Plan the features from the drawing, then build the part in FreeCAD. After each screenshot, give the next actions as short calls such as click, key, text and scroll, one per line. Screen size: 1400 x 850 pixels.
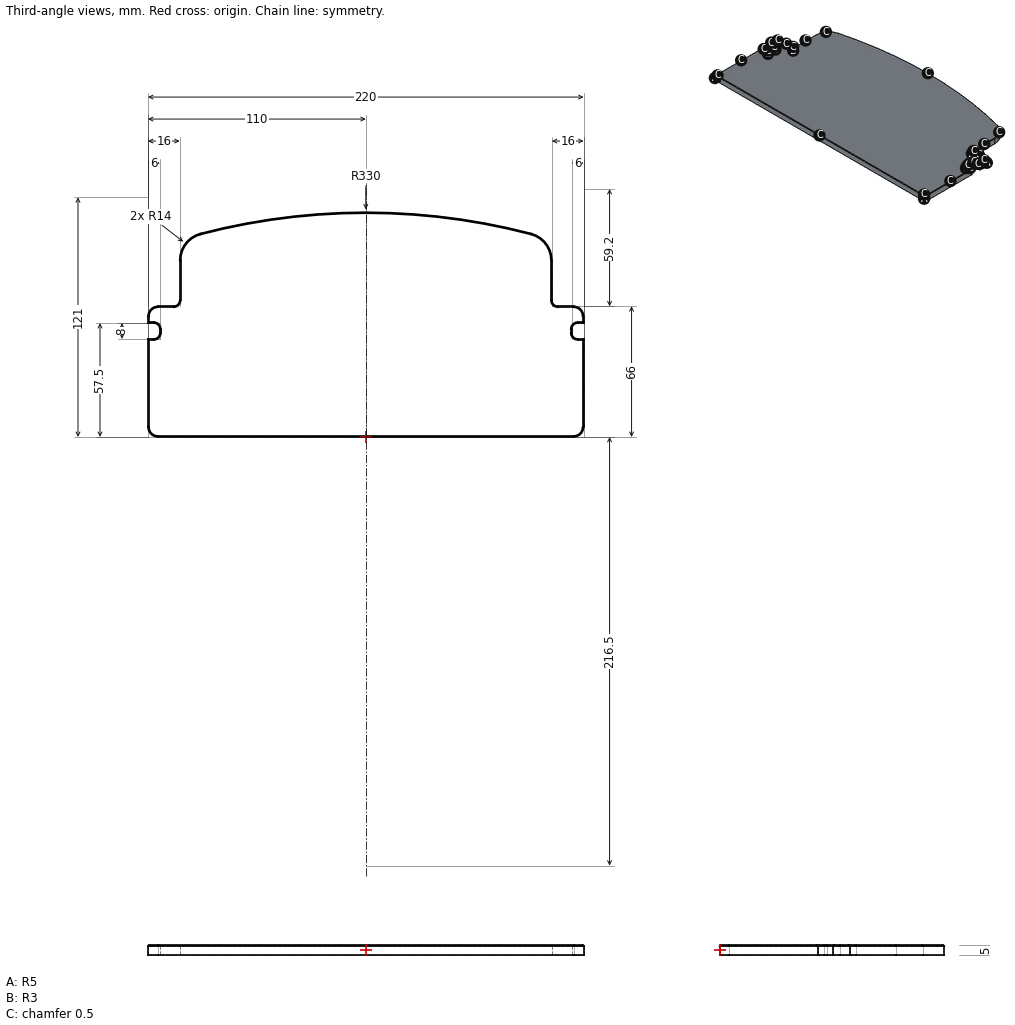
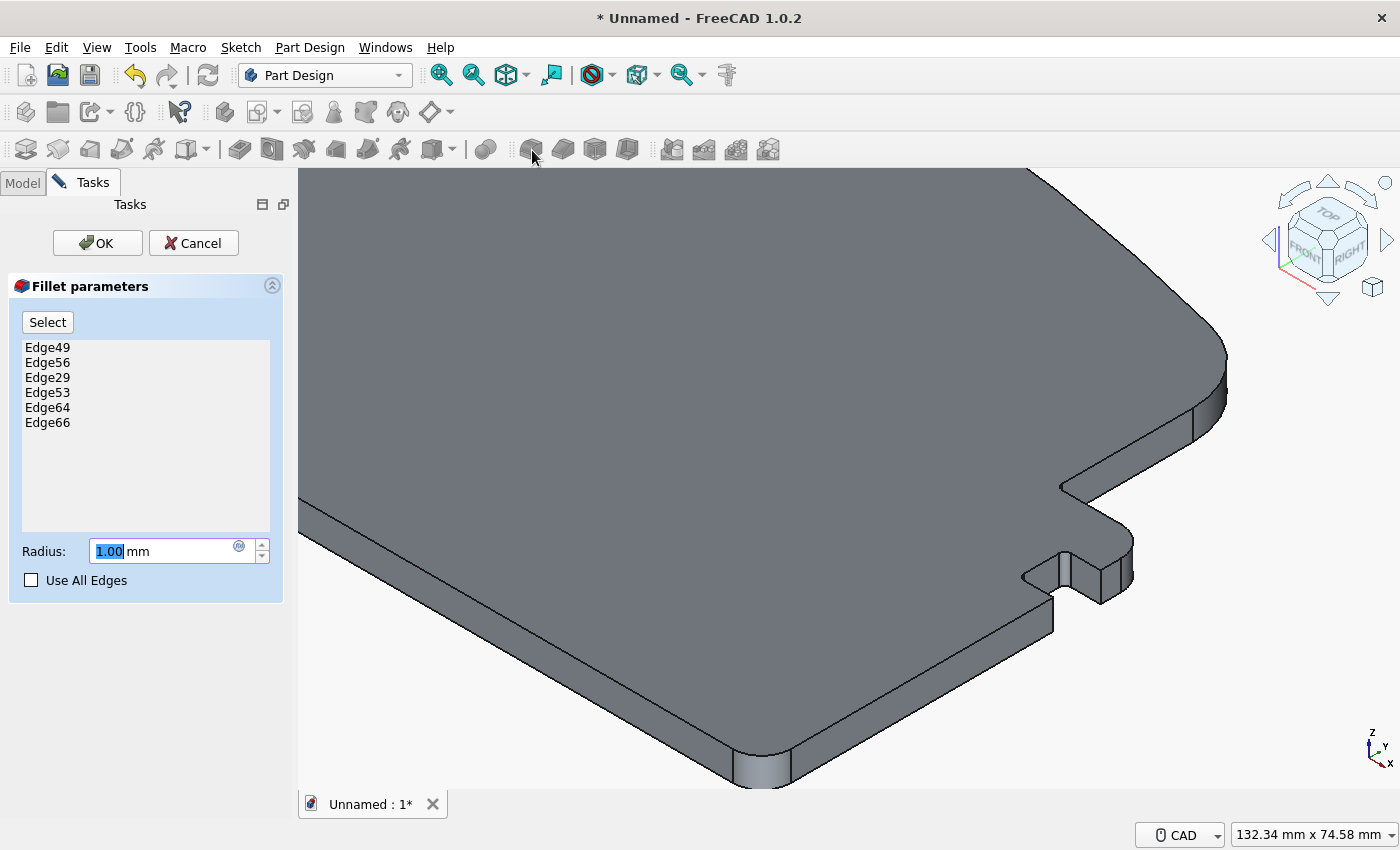
text(3)
key(Tab)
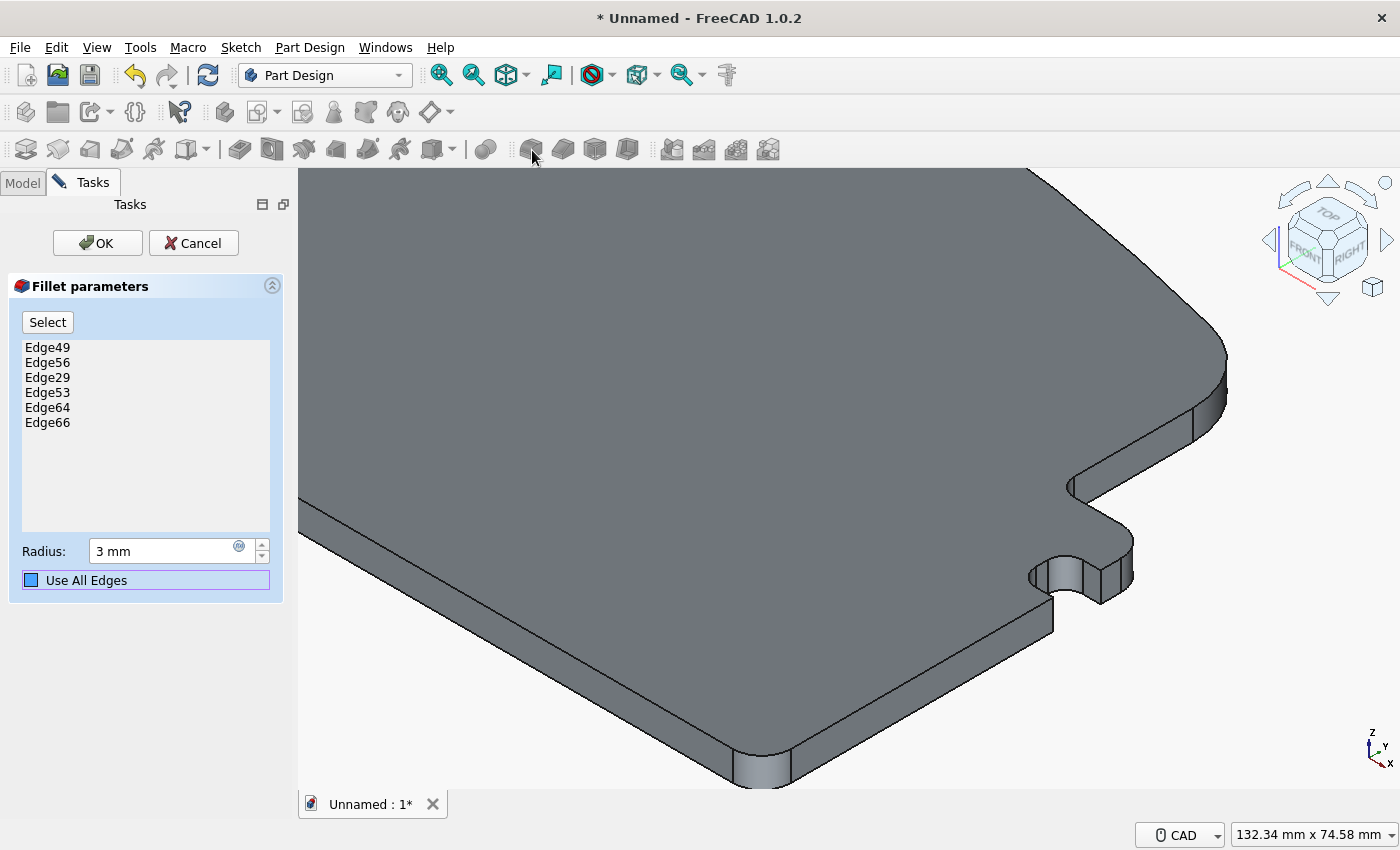
click(98, 243)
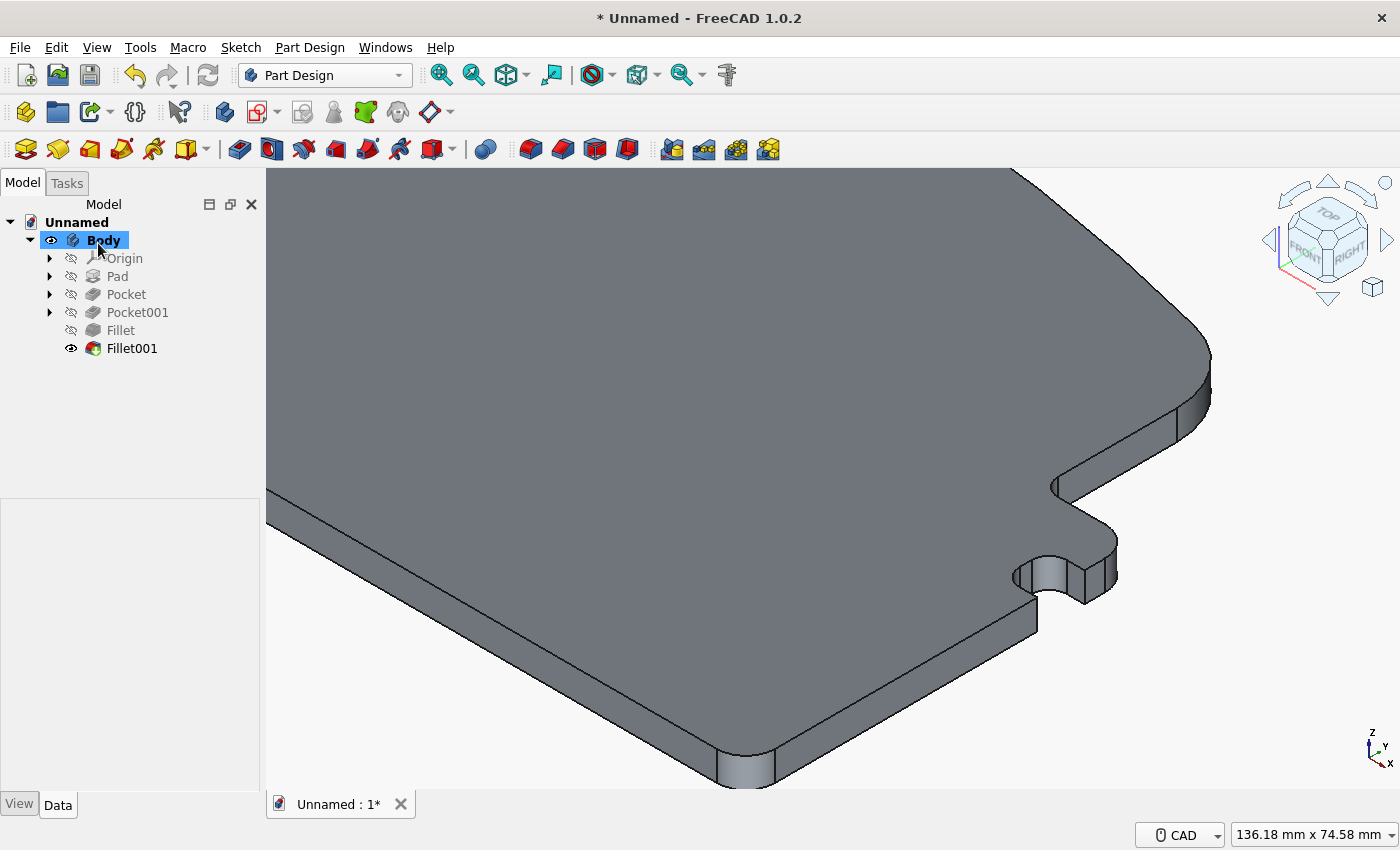
key(v)
key(f)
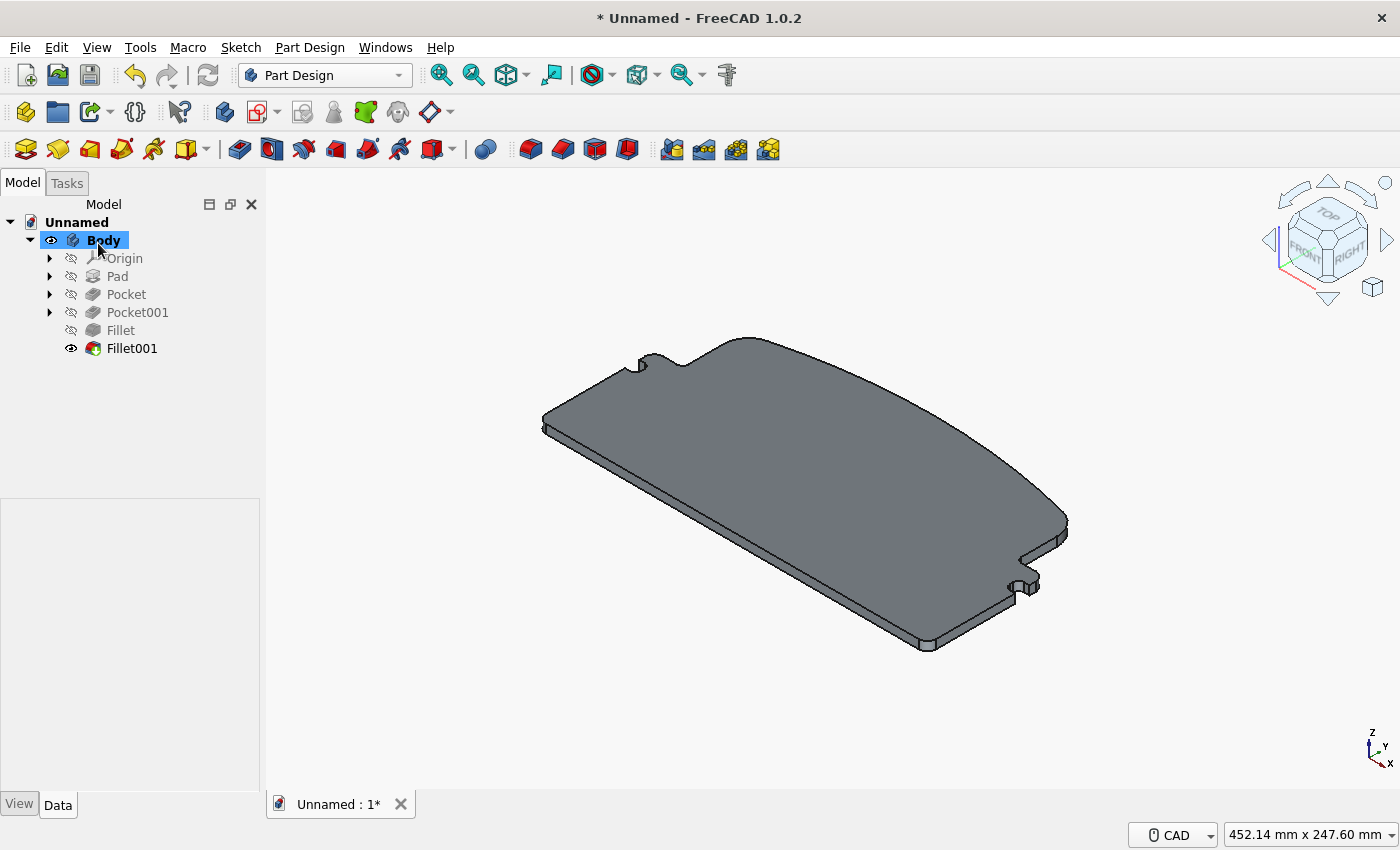
click(833, 472)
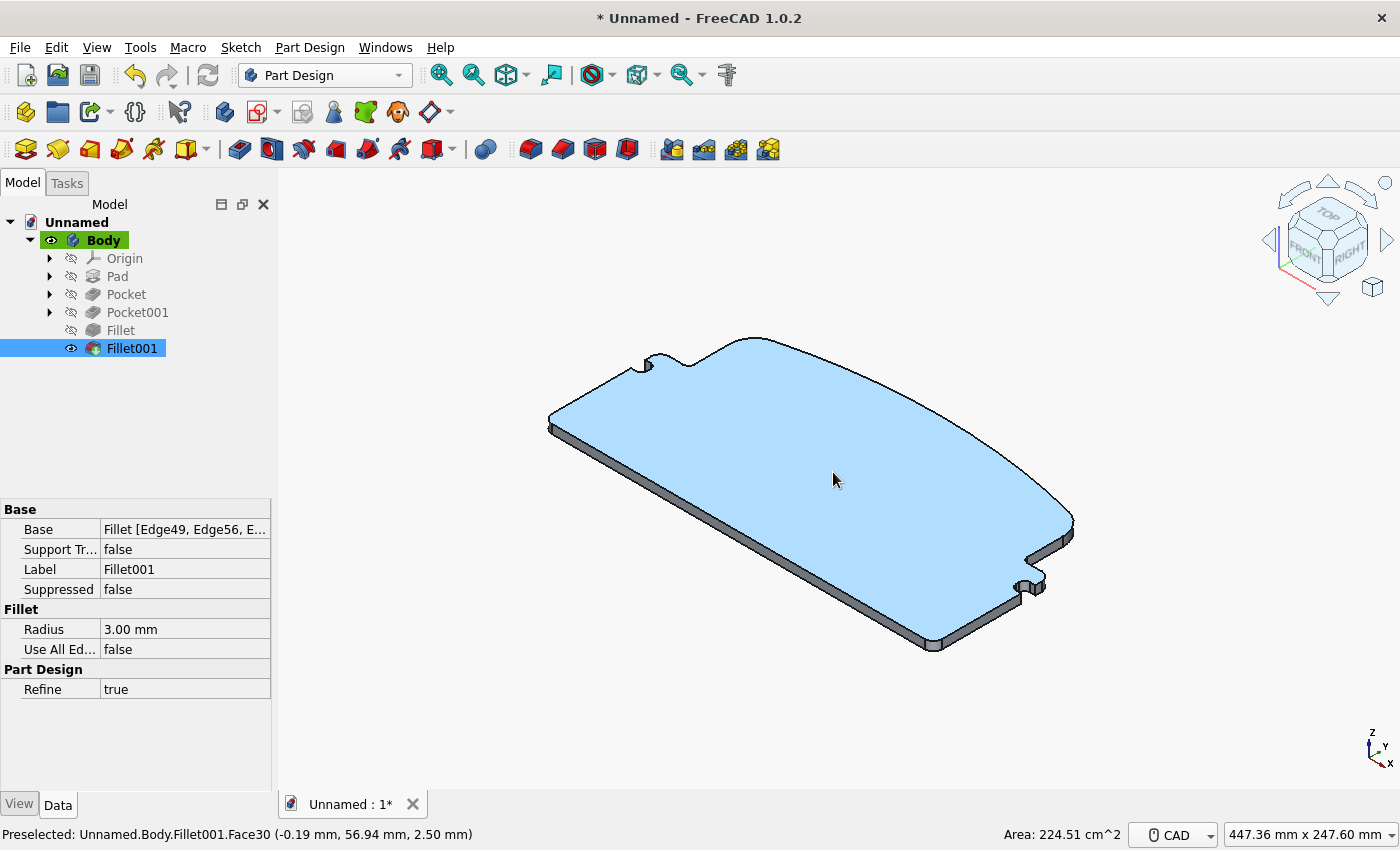
click(564, 150)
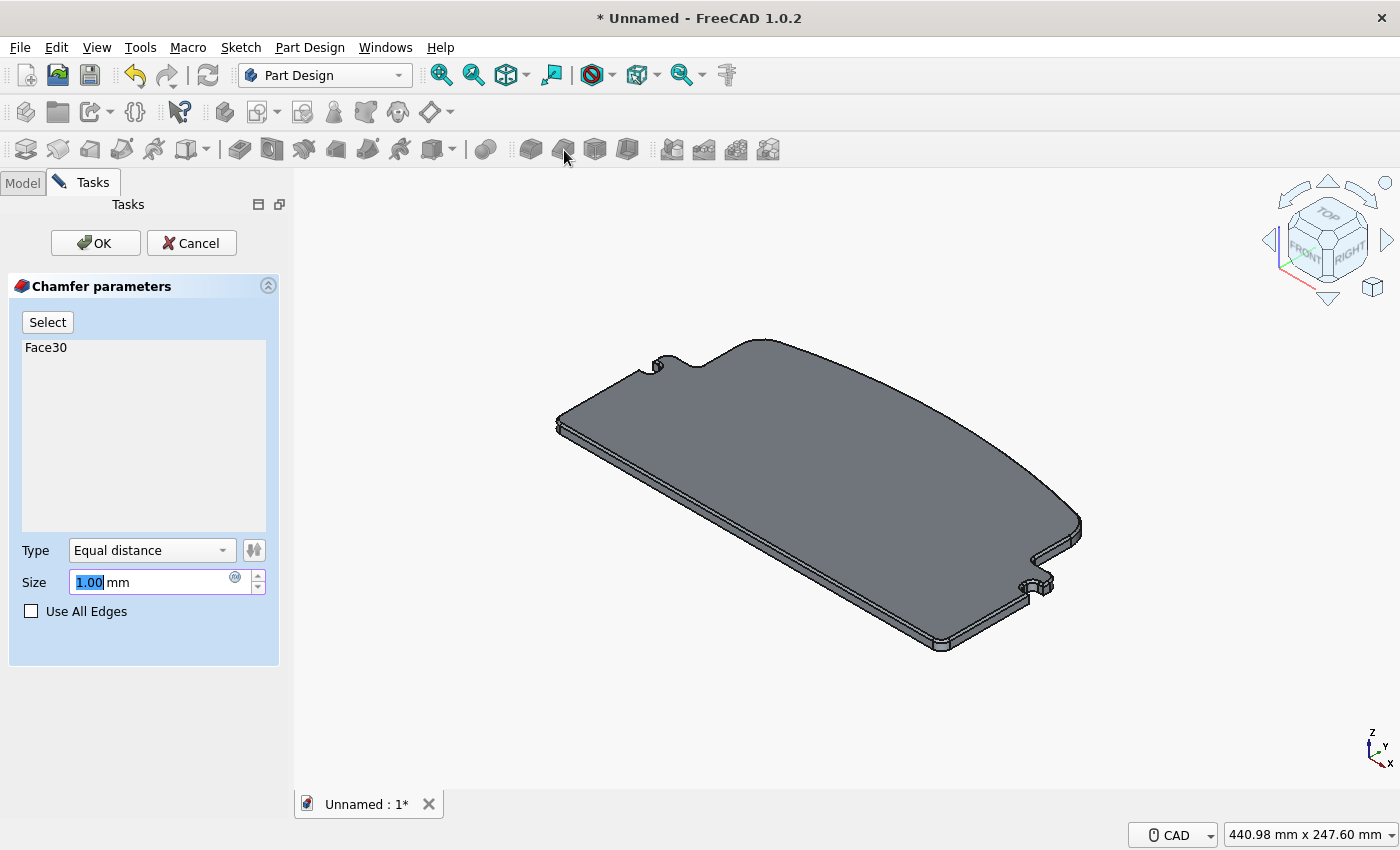
text(0.5)
key(Tab)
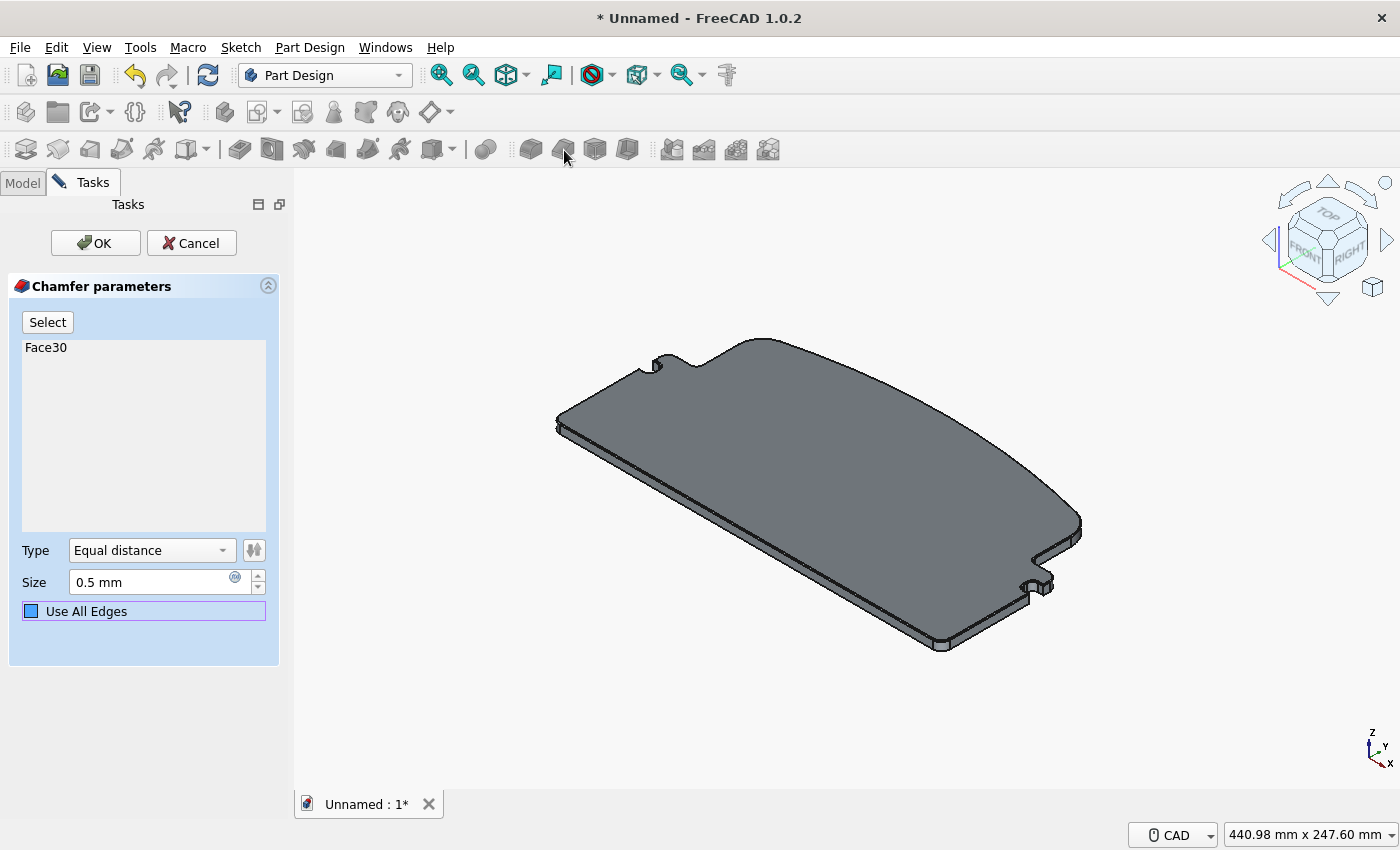
click(96, 243)